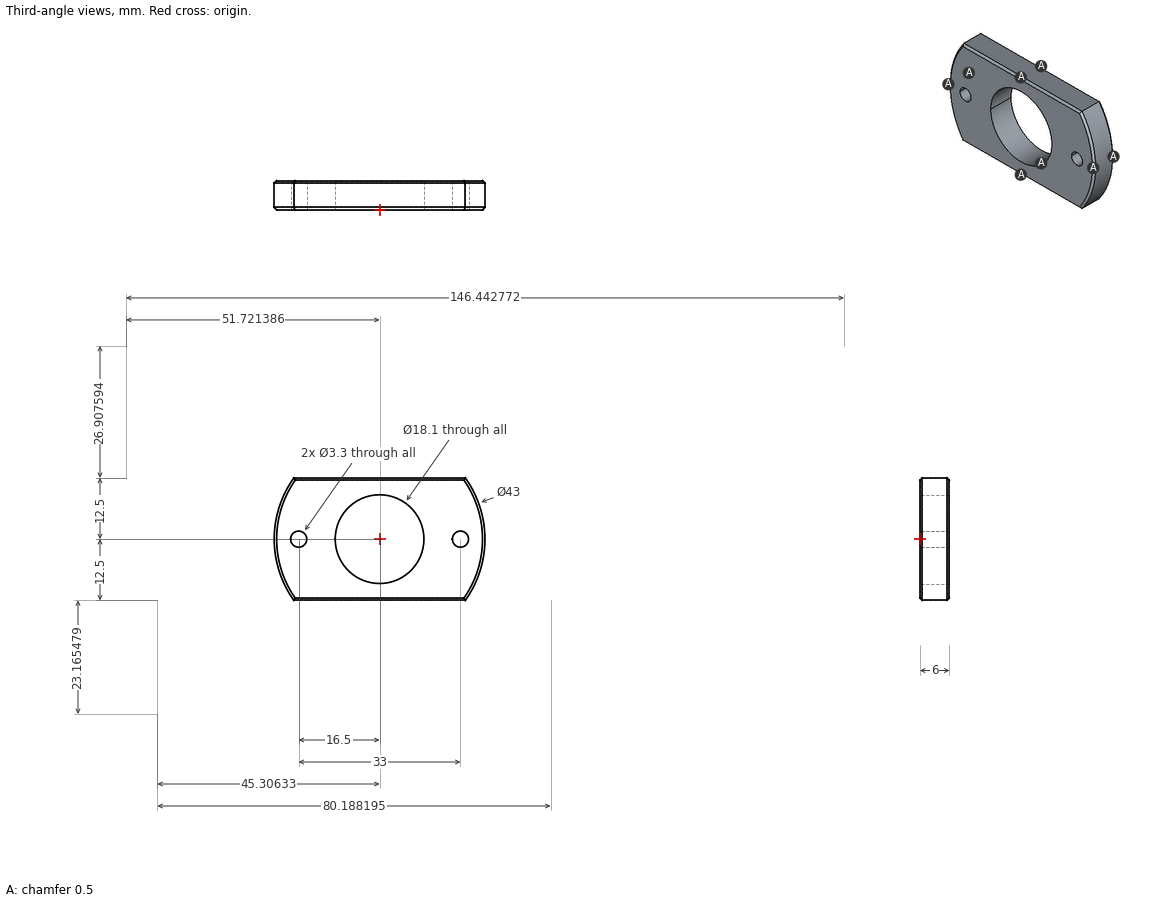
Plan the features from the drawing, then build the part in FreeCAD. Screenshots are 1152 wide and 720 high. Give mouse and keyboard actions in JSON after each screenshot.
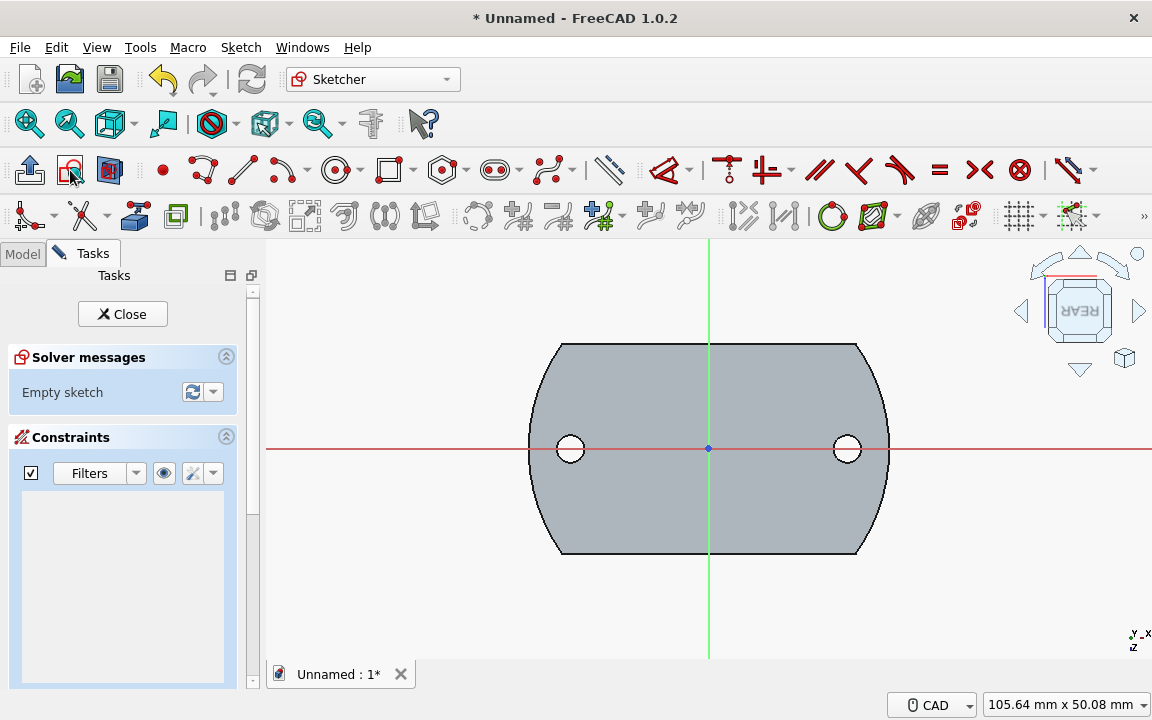
{"action": "scroll", "coordinate": [792, 449], "scroll_direction": "up", "scroll_amount": 3}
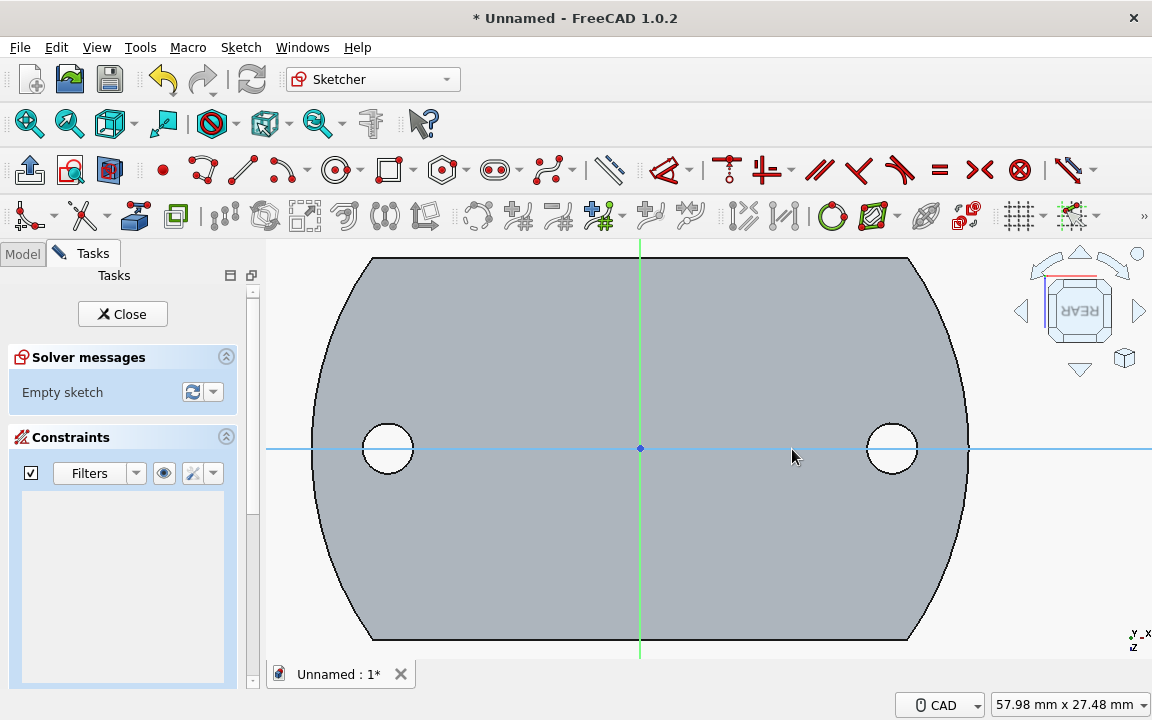
{"action": "left_click", "coordinate": [336, 170]}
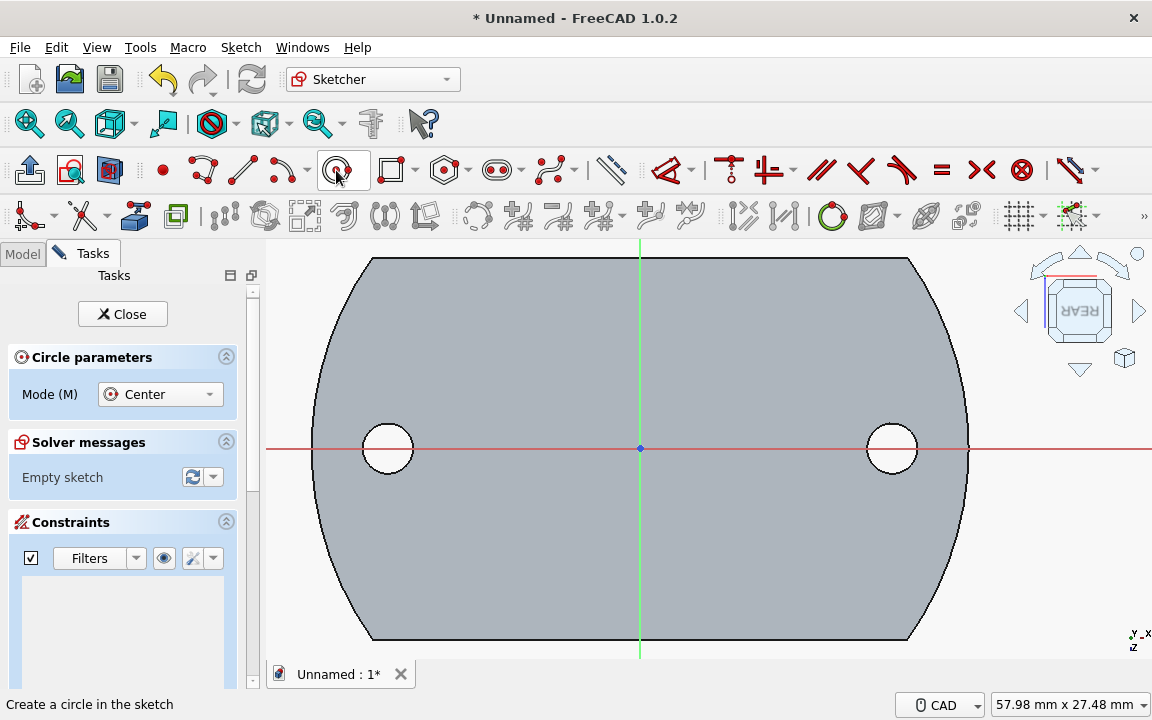
{"action": "left_click", "coordinate": [640, 449]}
{"action": "left_click", "coordinate": [738, 351]}
{"action": "key", "text": "Escape"}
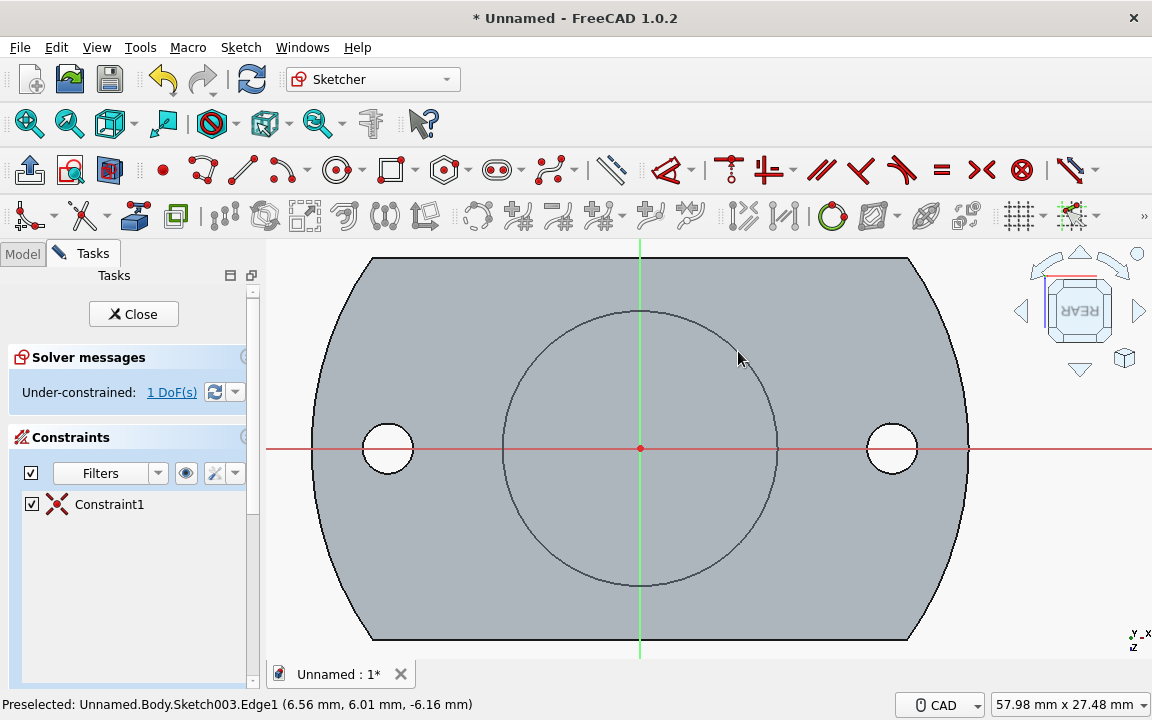
{"action": "left_click", "coordinate": [666, 170]}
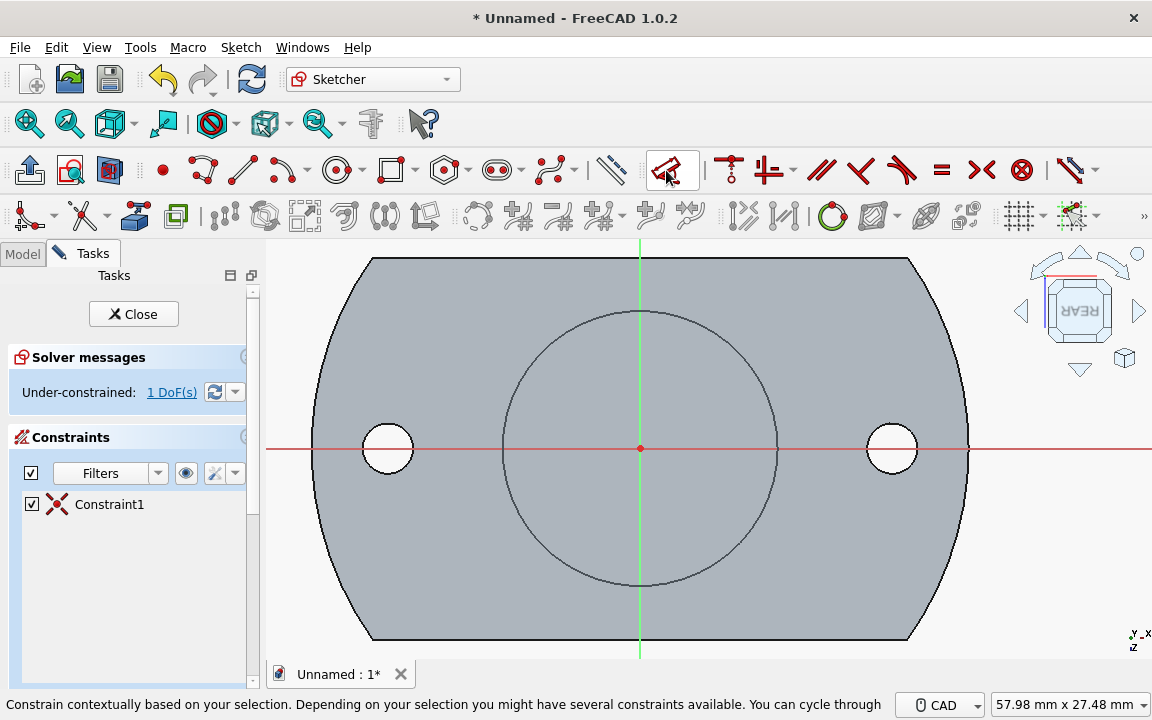
{"action": "left_click", "coordinate": [737, 351]}
{"action": "left_click", "coordinate": [760, 328]}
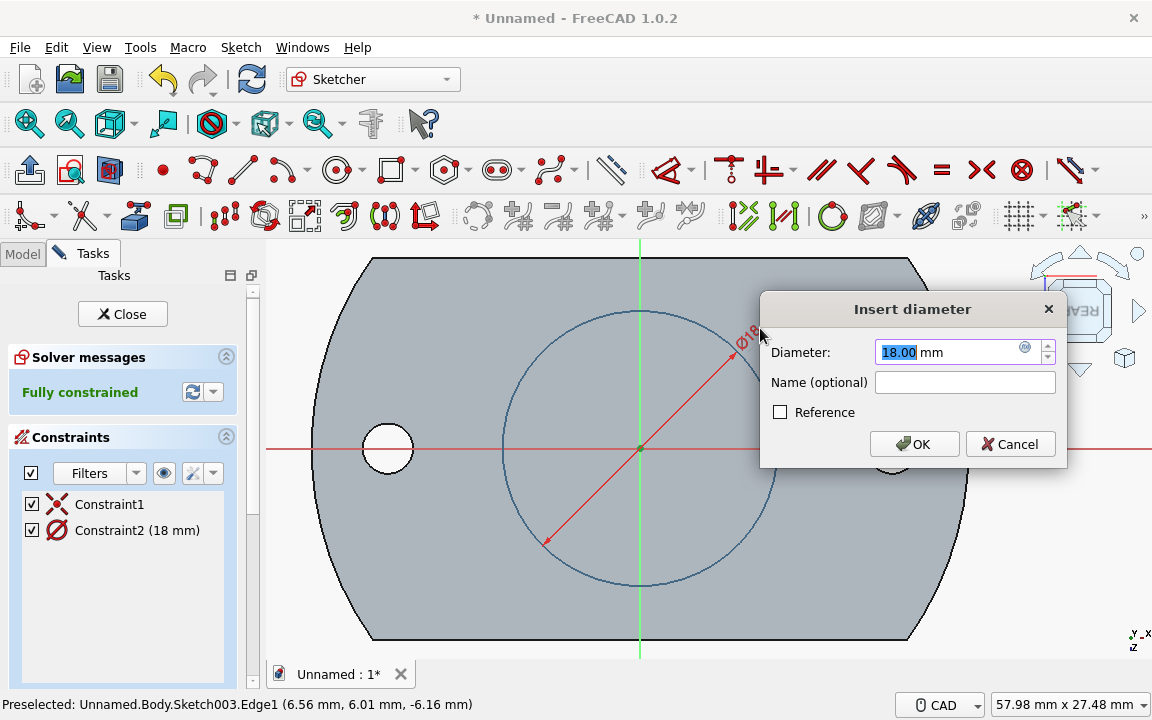
{"action": "type", "text": "18.1"}
{"action": "key", "text": "Return"}
{"action": "key", "text": "Escape"}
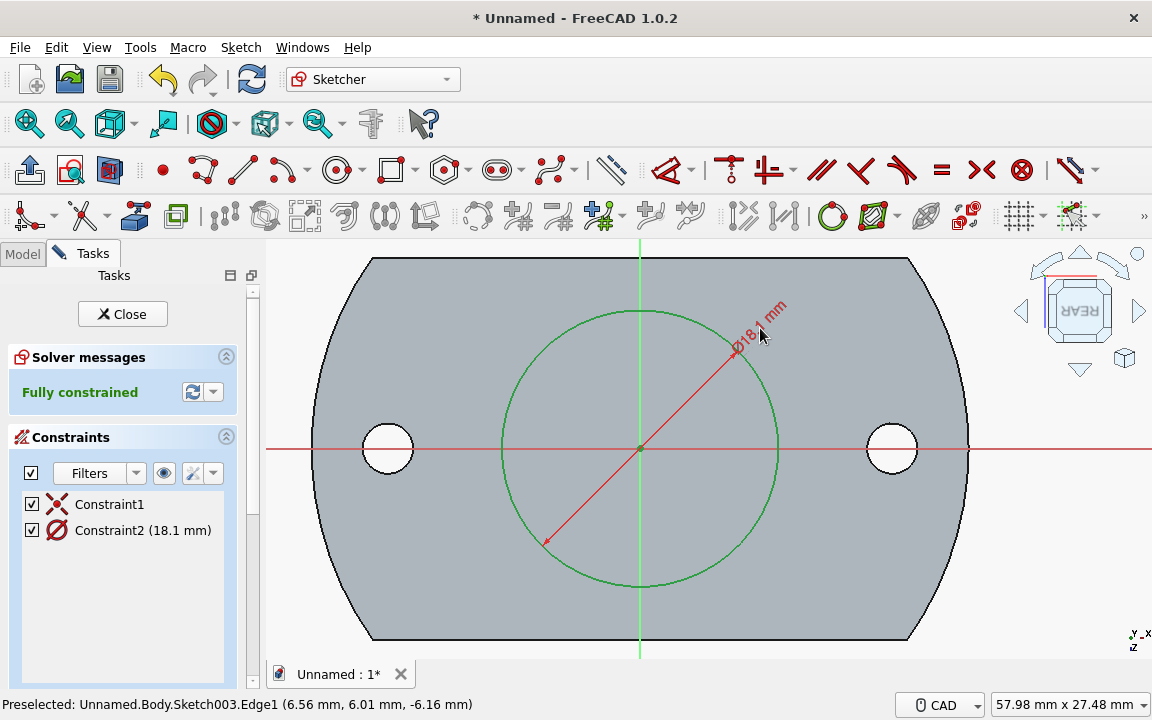
{"action": "left_click", "coordinate": [123, 314]}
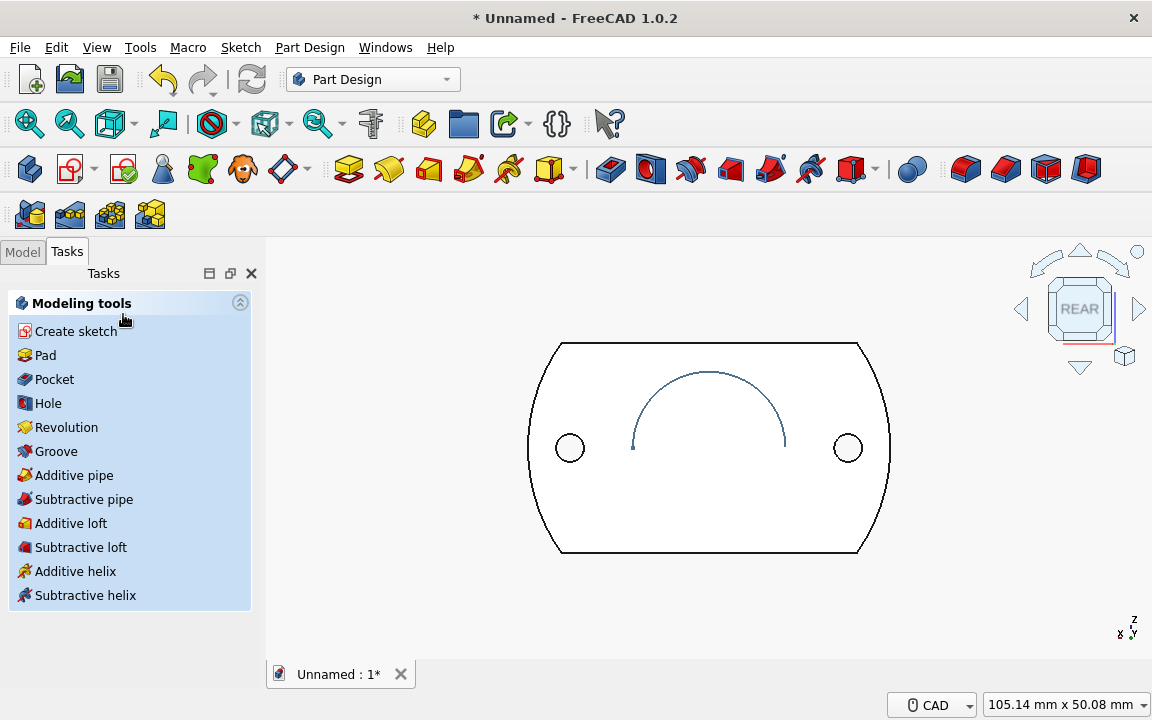
{"action": "left_click", "coordinate": [652, 170]}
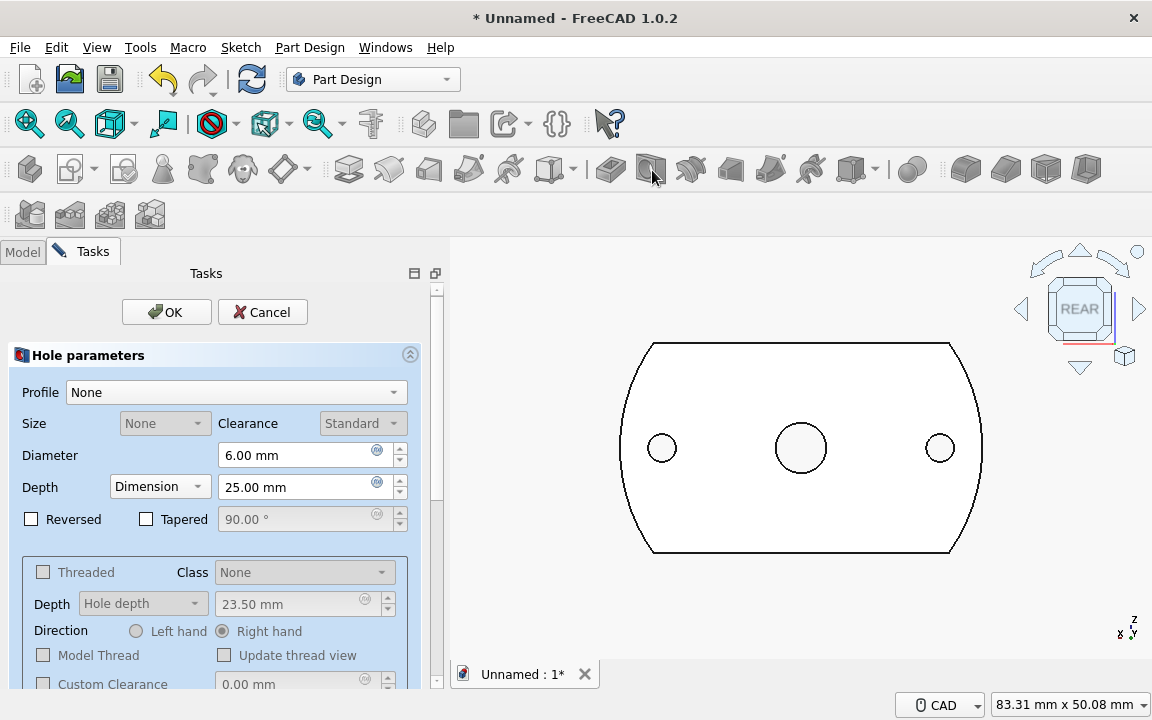
{"action": "triple_click", "coordinate": [305, 455]}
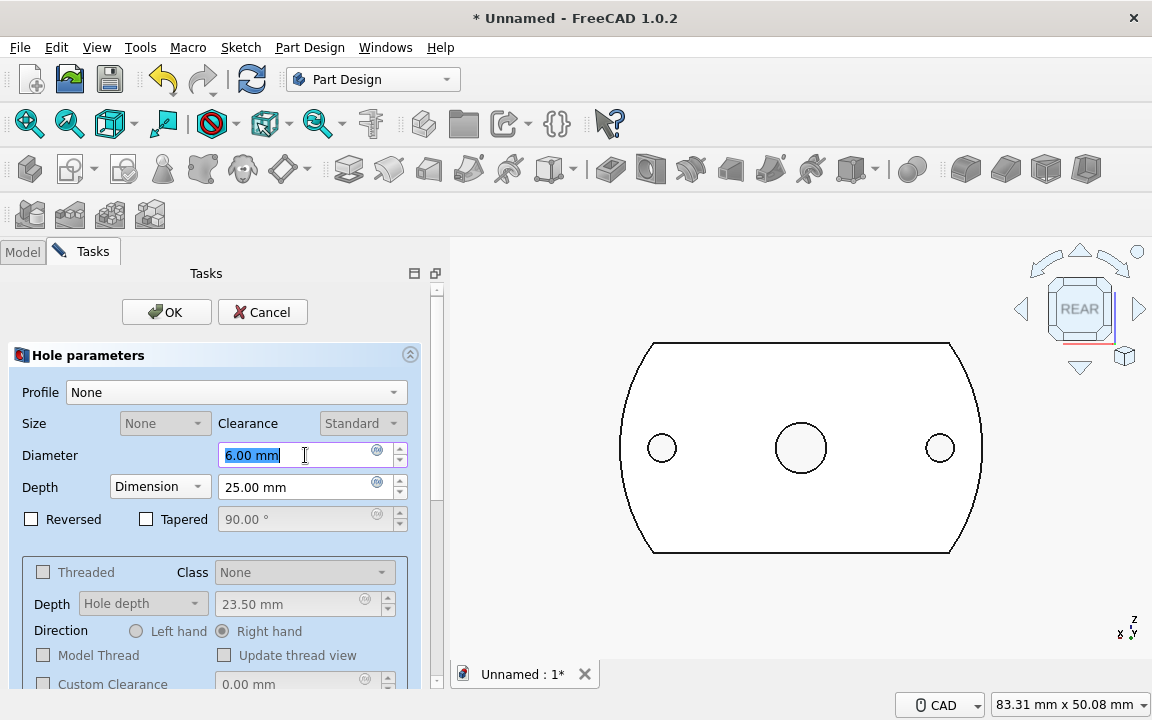
{"action": "type", "text": "18.1"}
{"action": "key", "text": "Tab"}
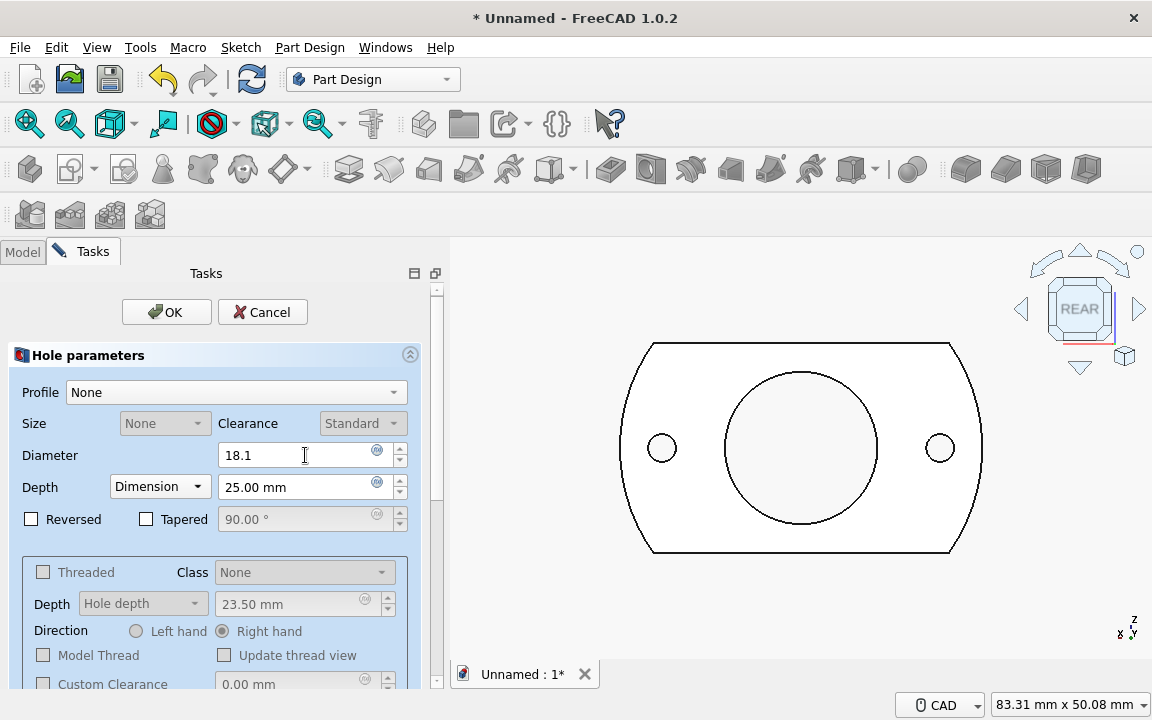
{"action": "left_click", "coordinate": [161, 486]}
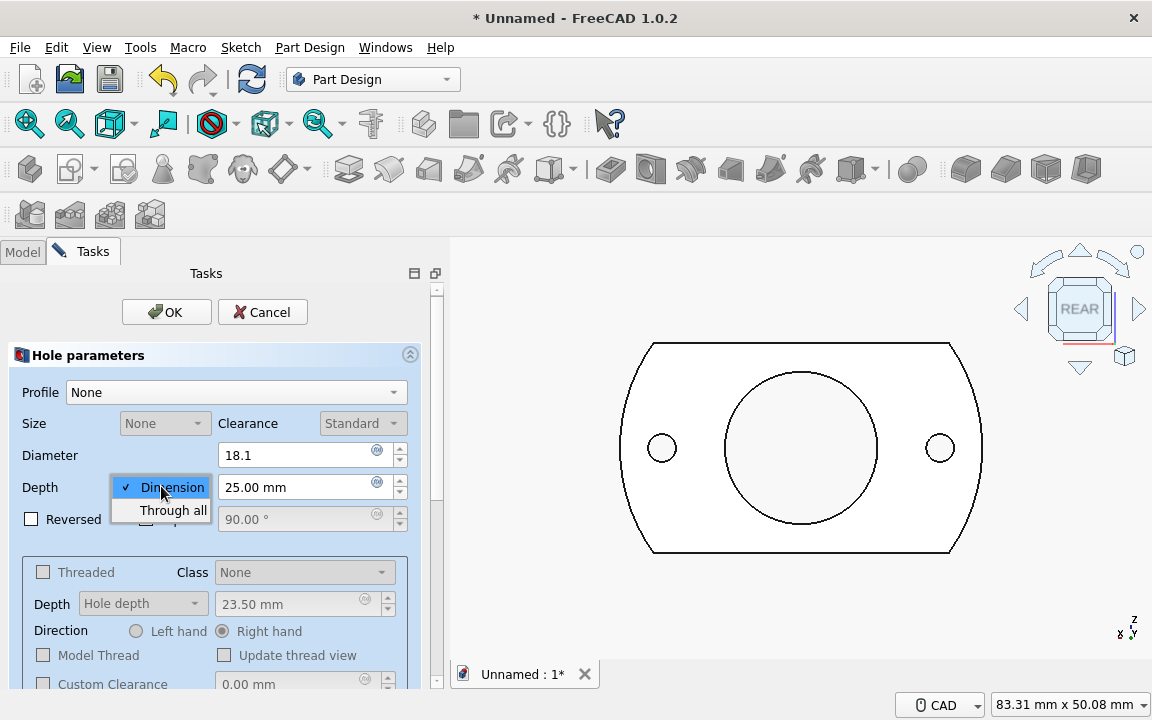
{"action": "left_click", "coordinate": [160, 510]}